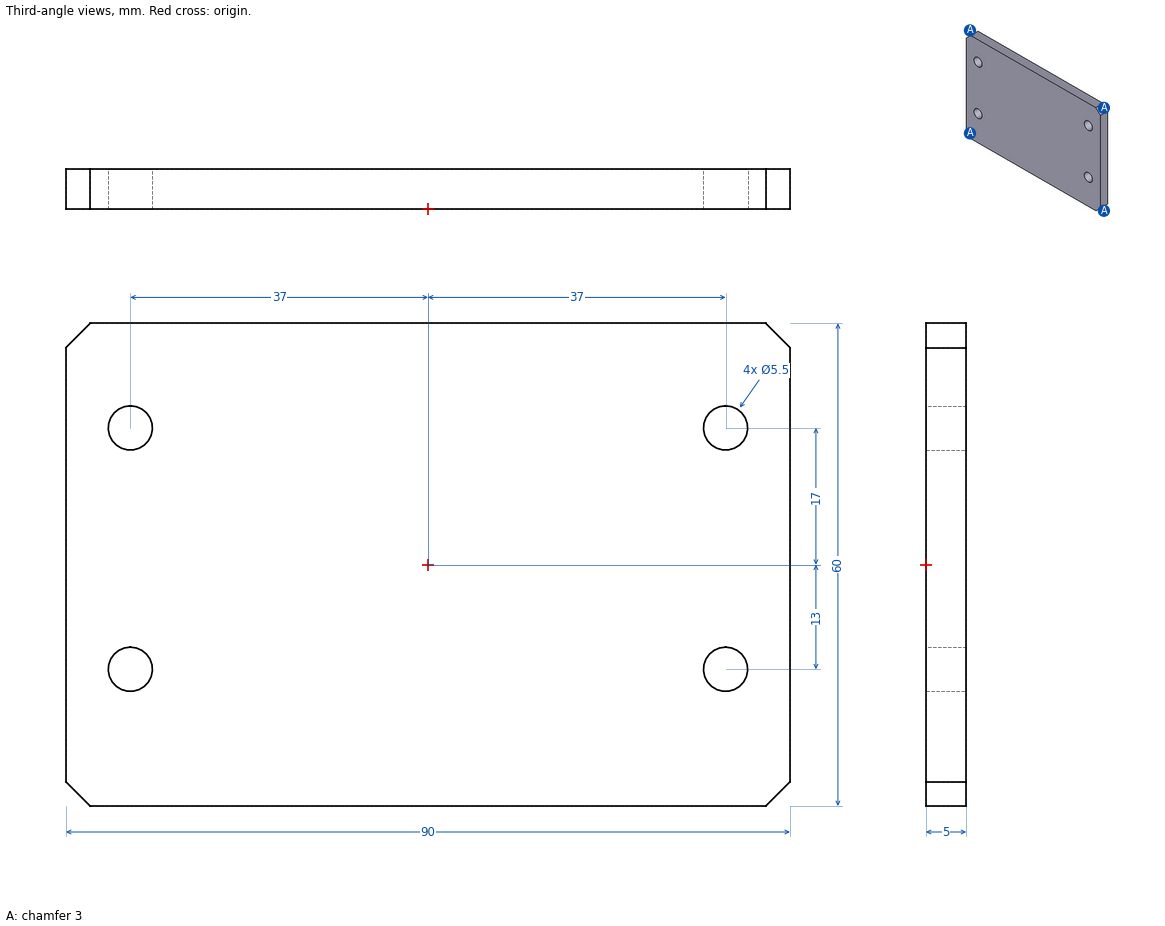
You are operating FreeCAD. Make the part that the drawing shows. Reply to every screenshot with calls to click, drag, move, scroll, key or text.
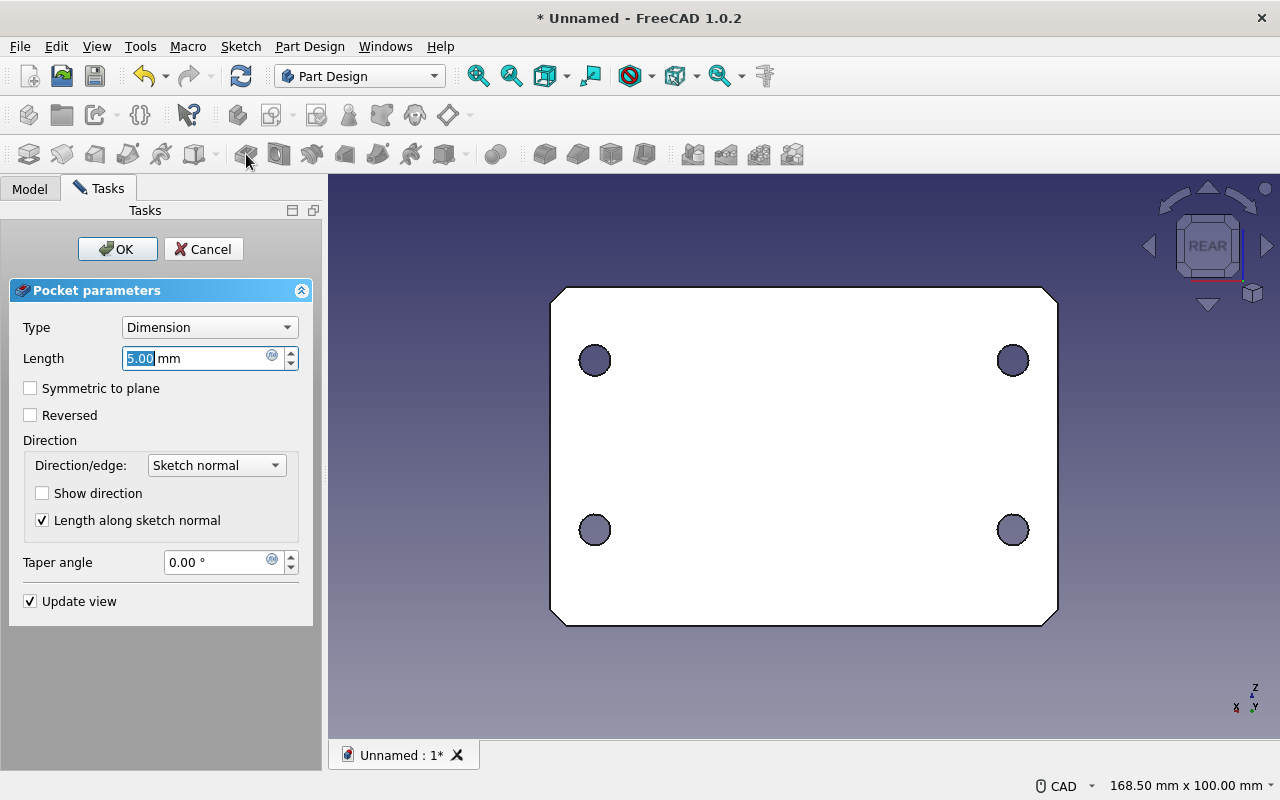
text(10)
key(Tab)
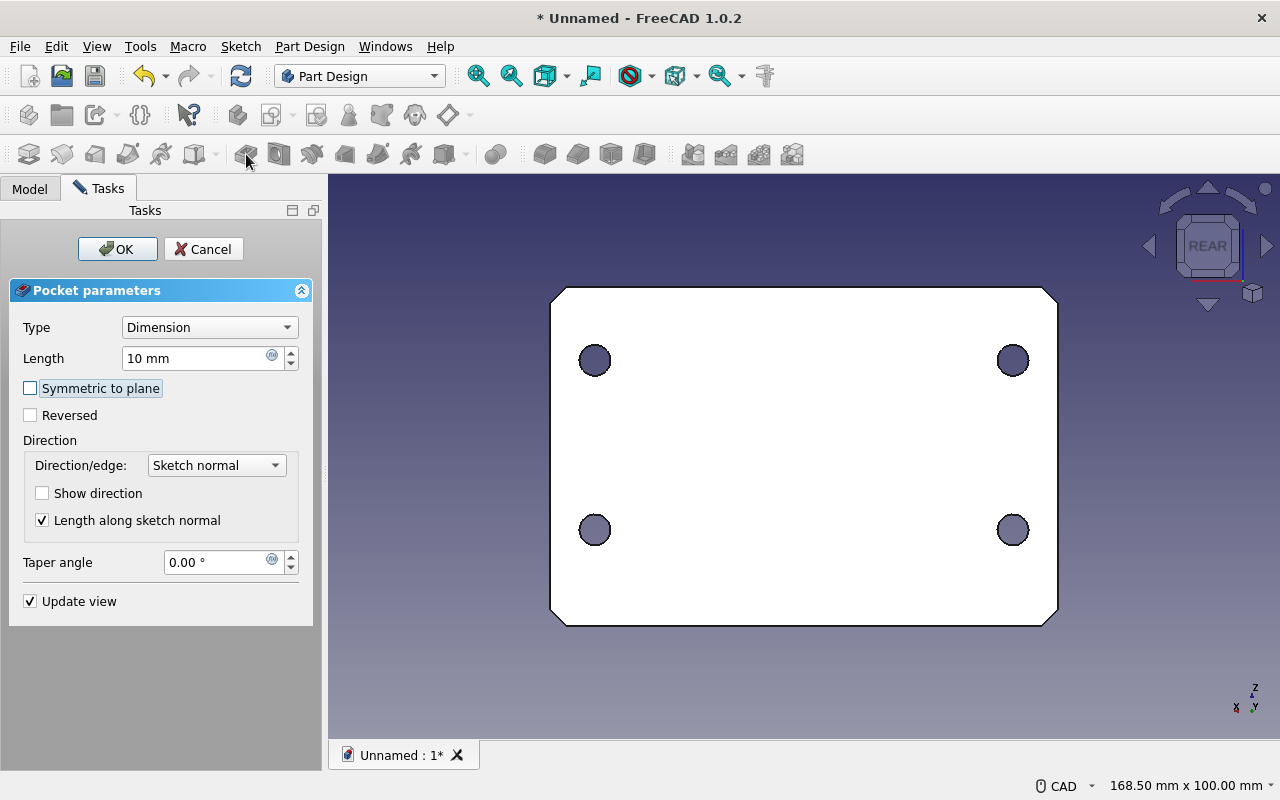
click(118, 249)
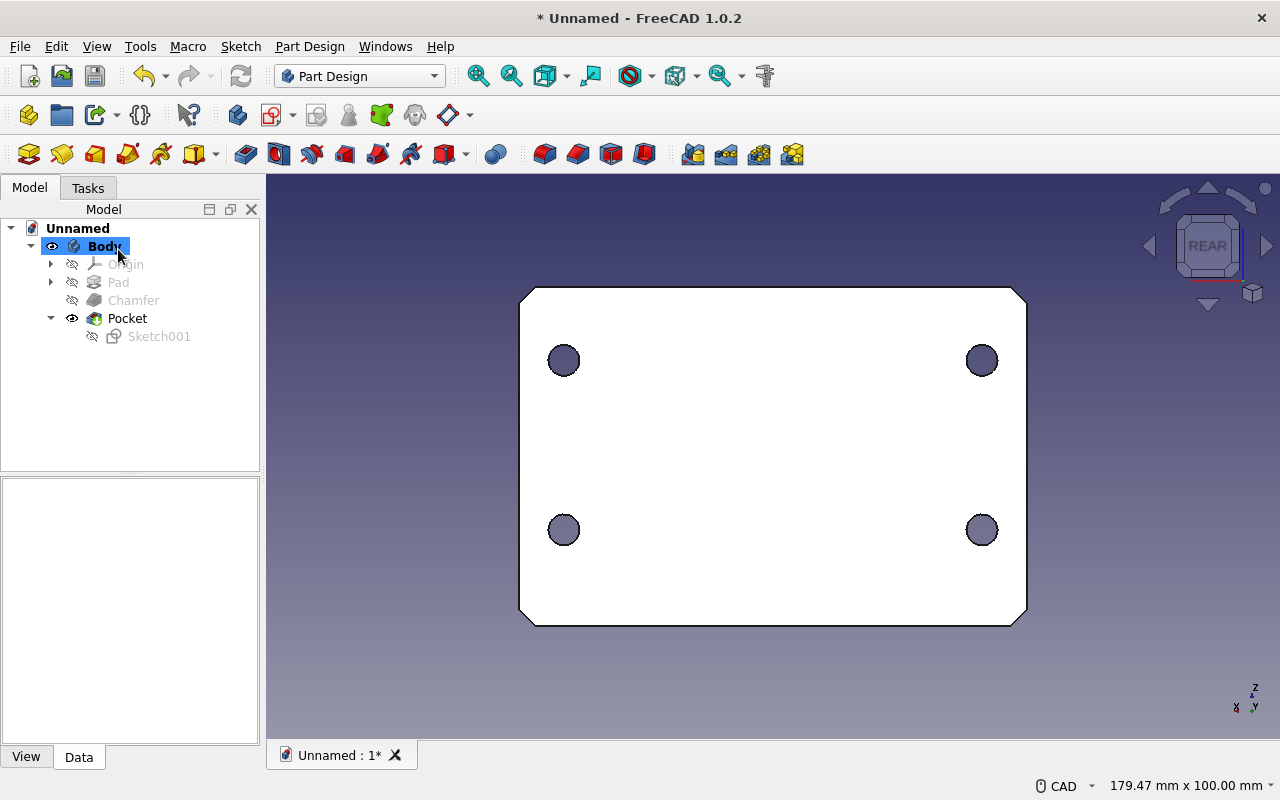
key(0)